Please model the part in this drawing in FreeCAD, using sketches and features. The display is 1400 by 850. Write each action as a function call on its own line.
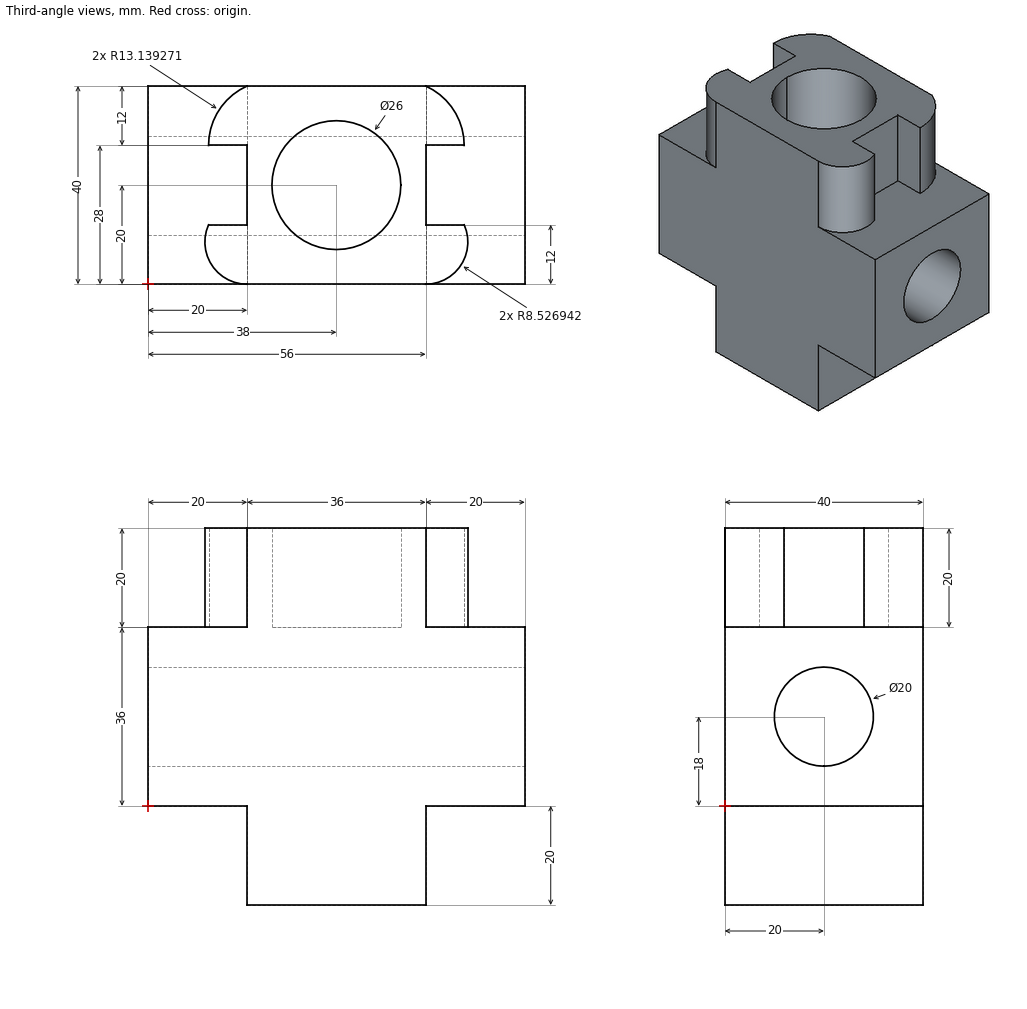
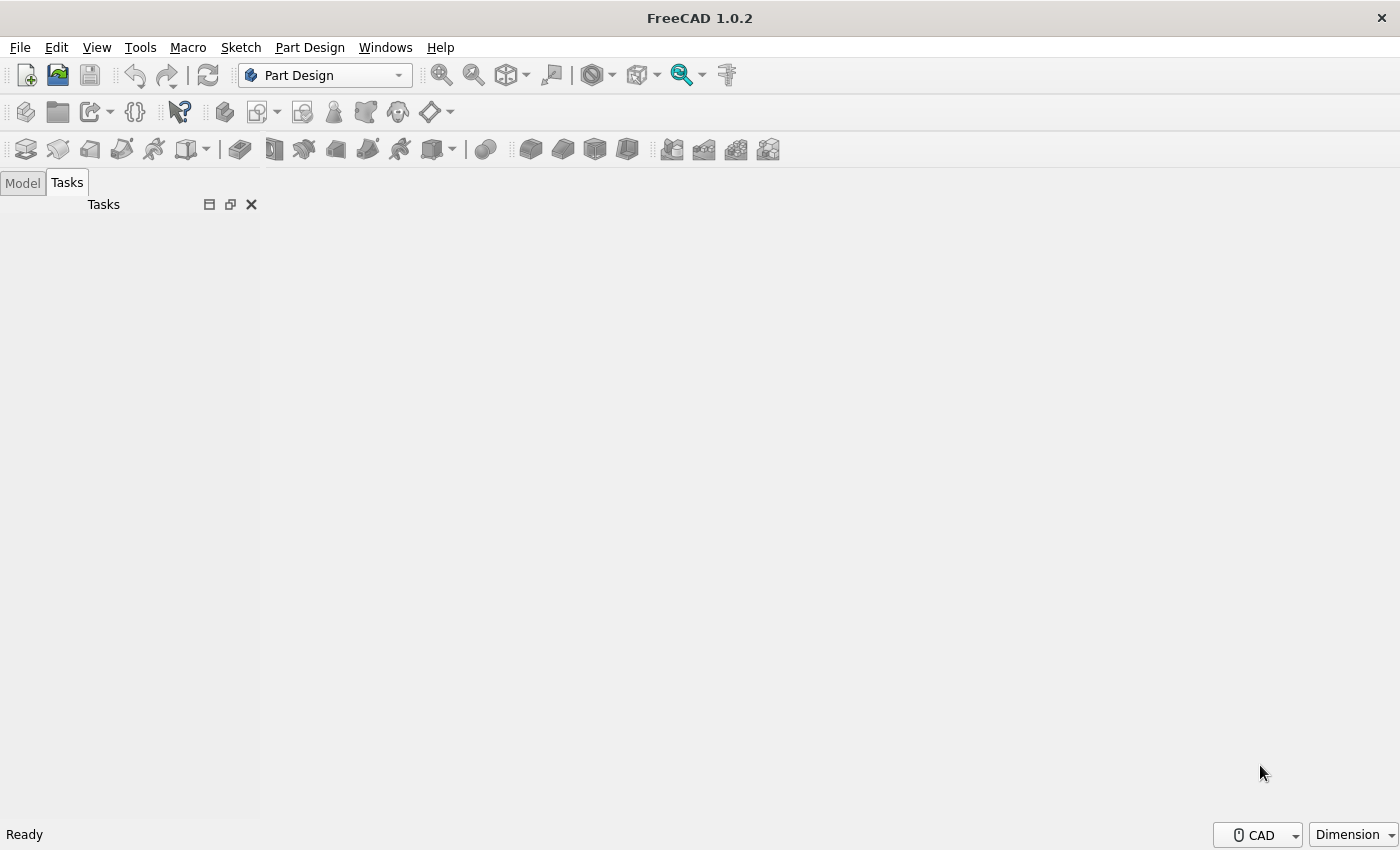
click(1032, 76)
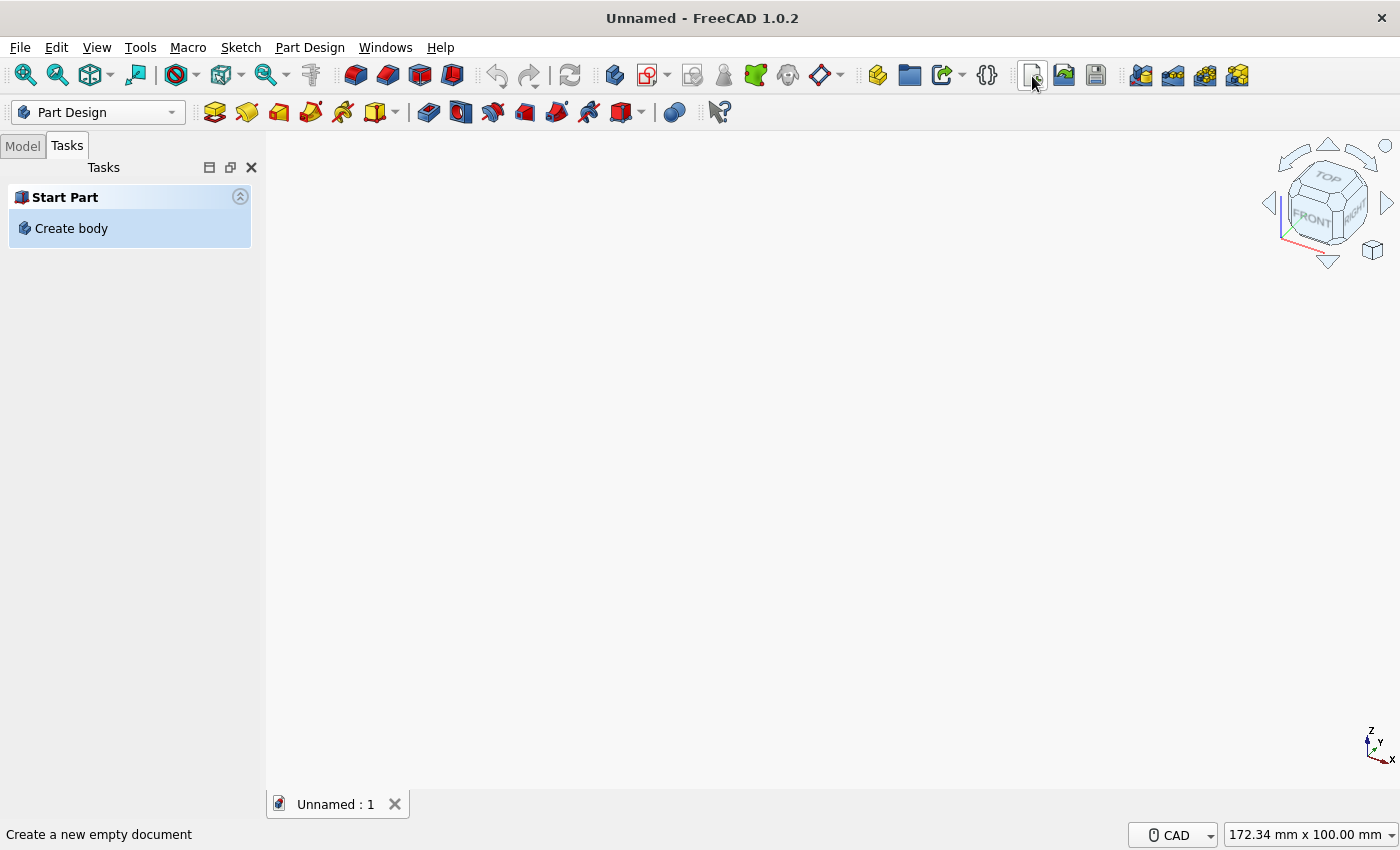
click(648, 76)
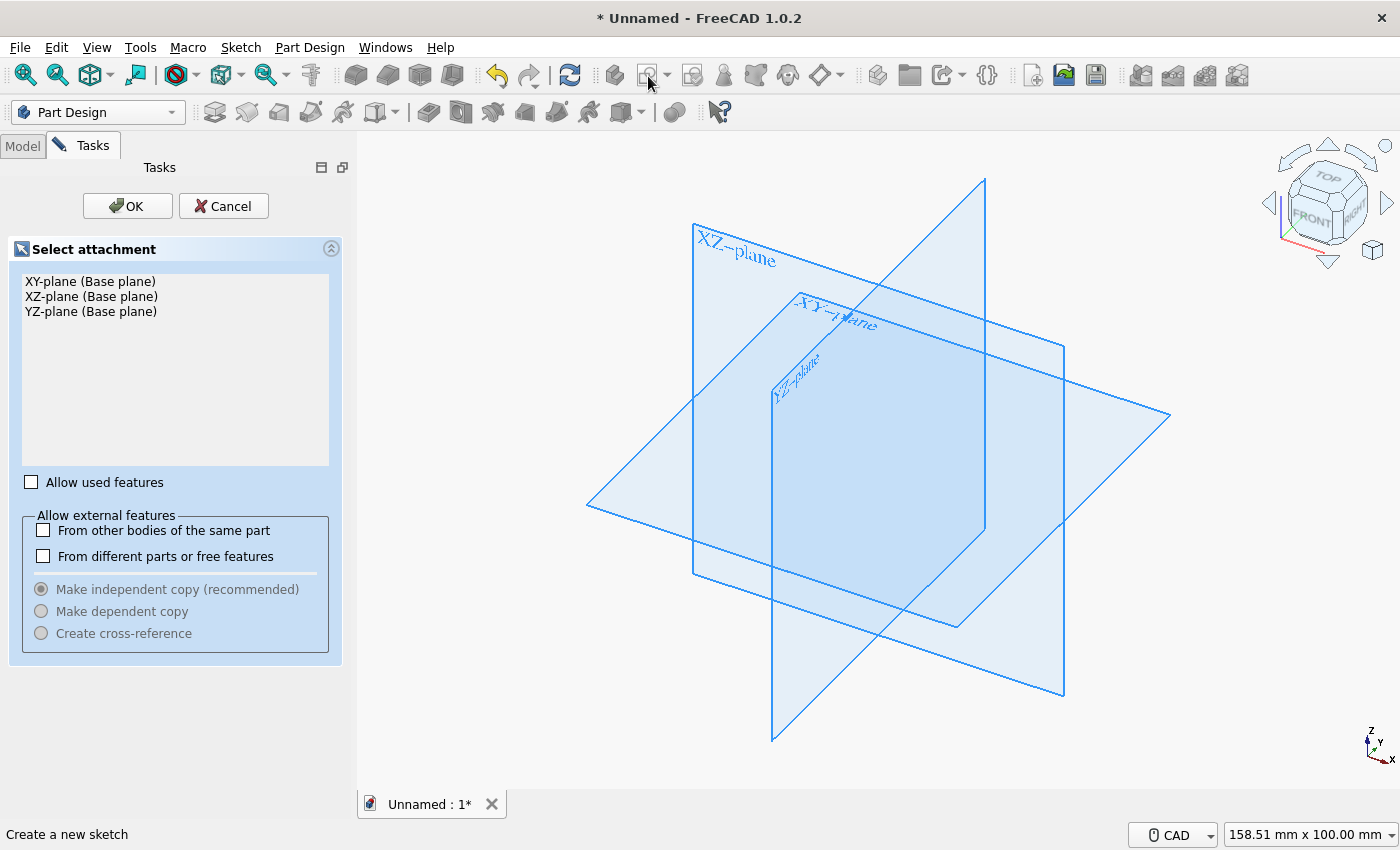
click(82, 296)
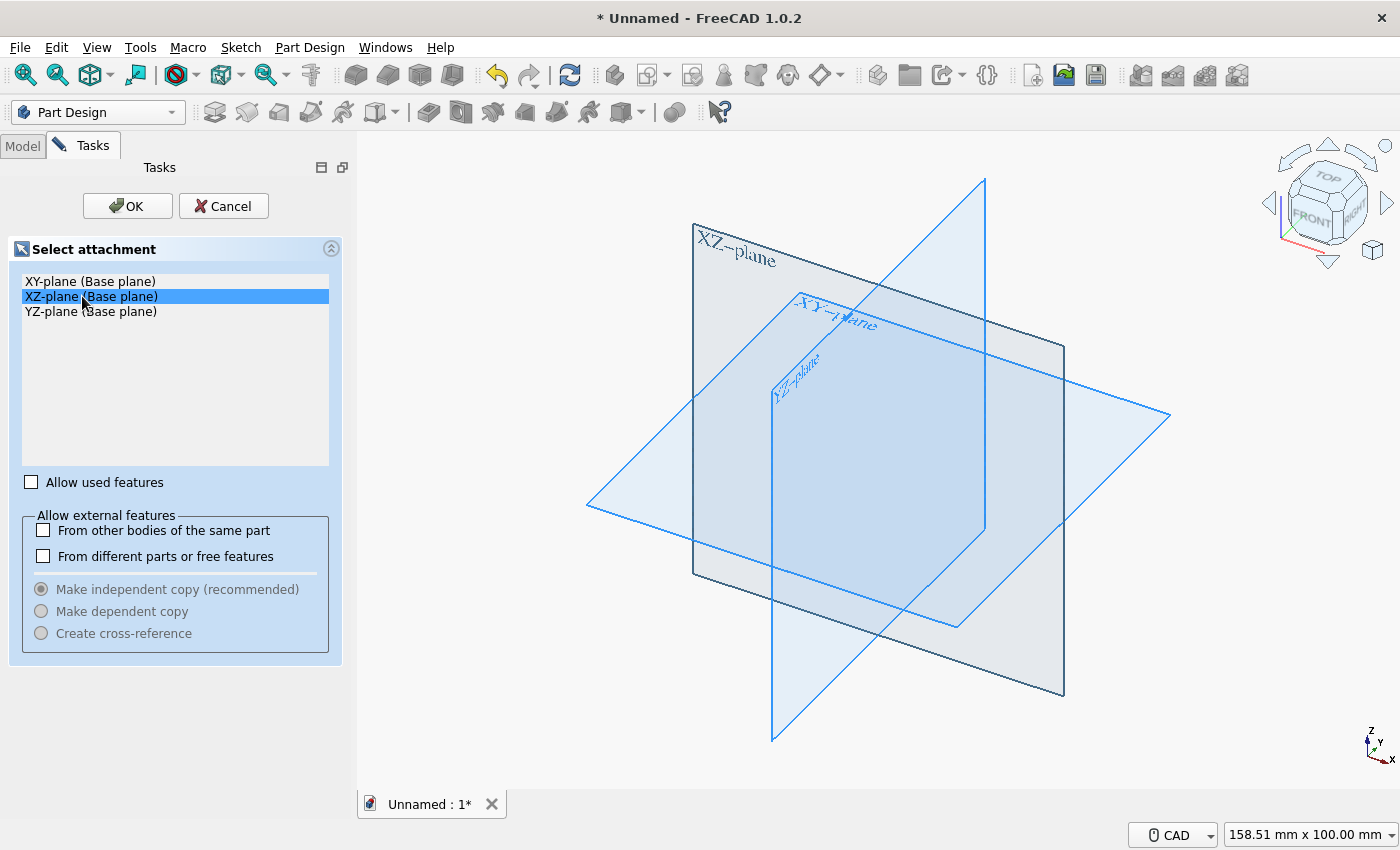
click(128, 206)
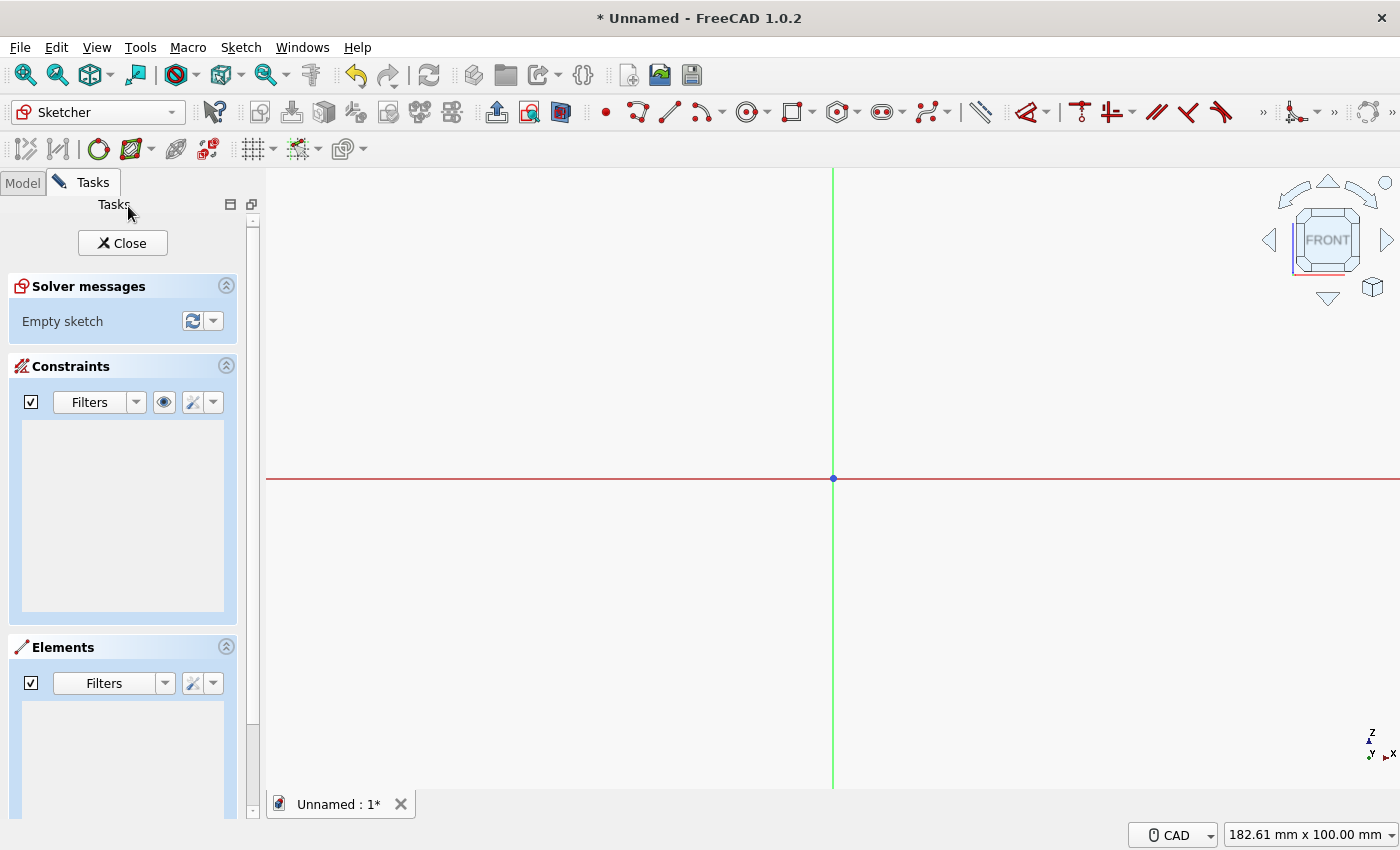
scroll(294, 761, down, 1)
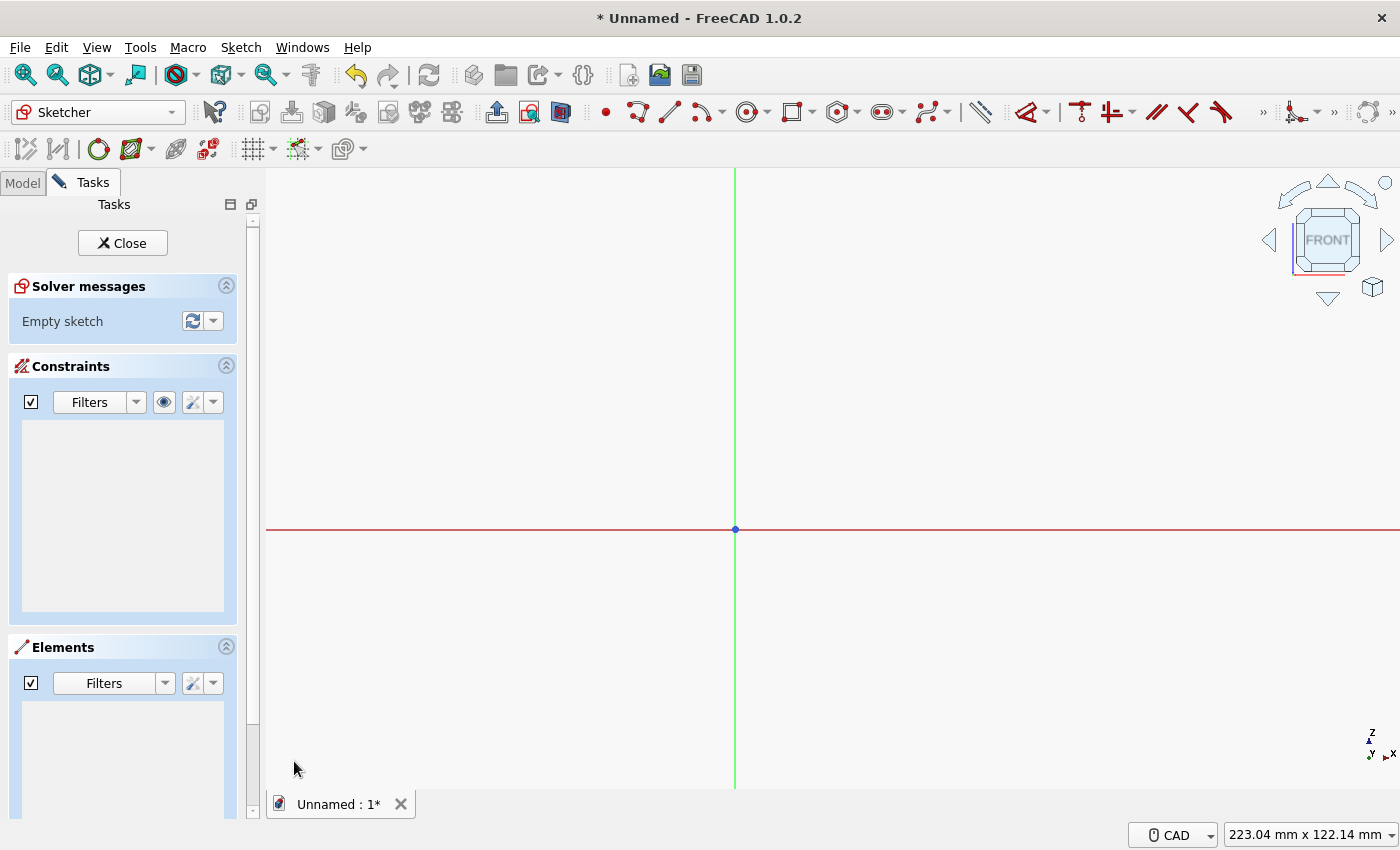
click(638, 112)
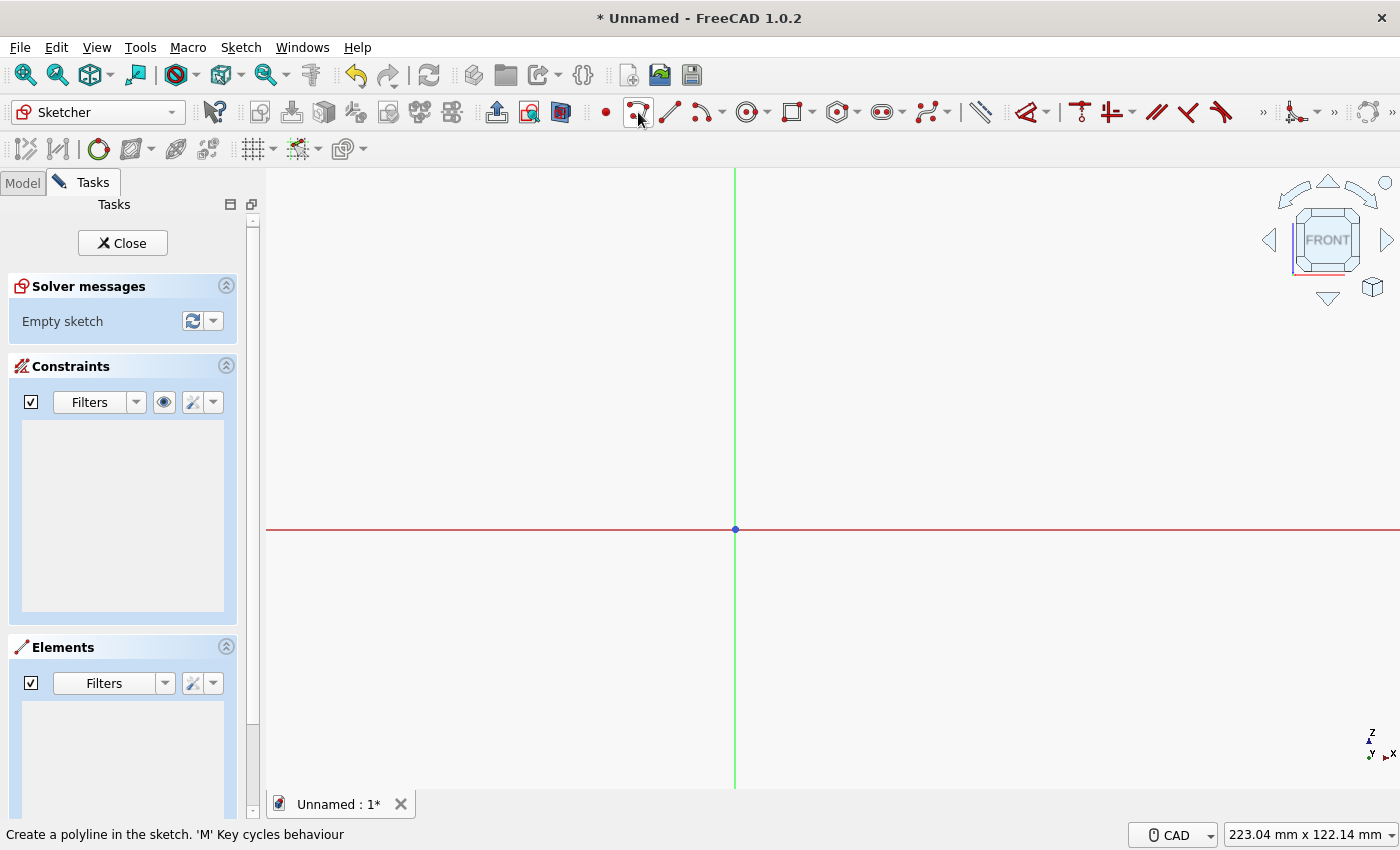
click(735, 530)
click(744, 347)
click(837, 347)
click(837, 245)
click(1020, 245)
click(1020, 347)
click(1122, 347)
click(1122, 530)
click(1020, 521)
click(1020, 632)
click(837, 632)
click(837, 521)
click(735, 530)
key(Escape)
key(Escape)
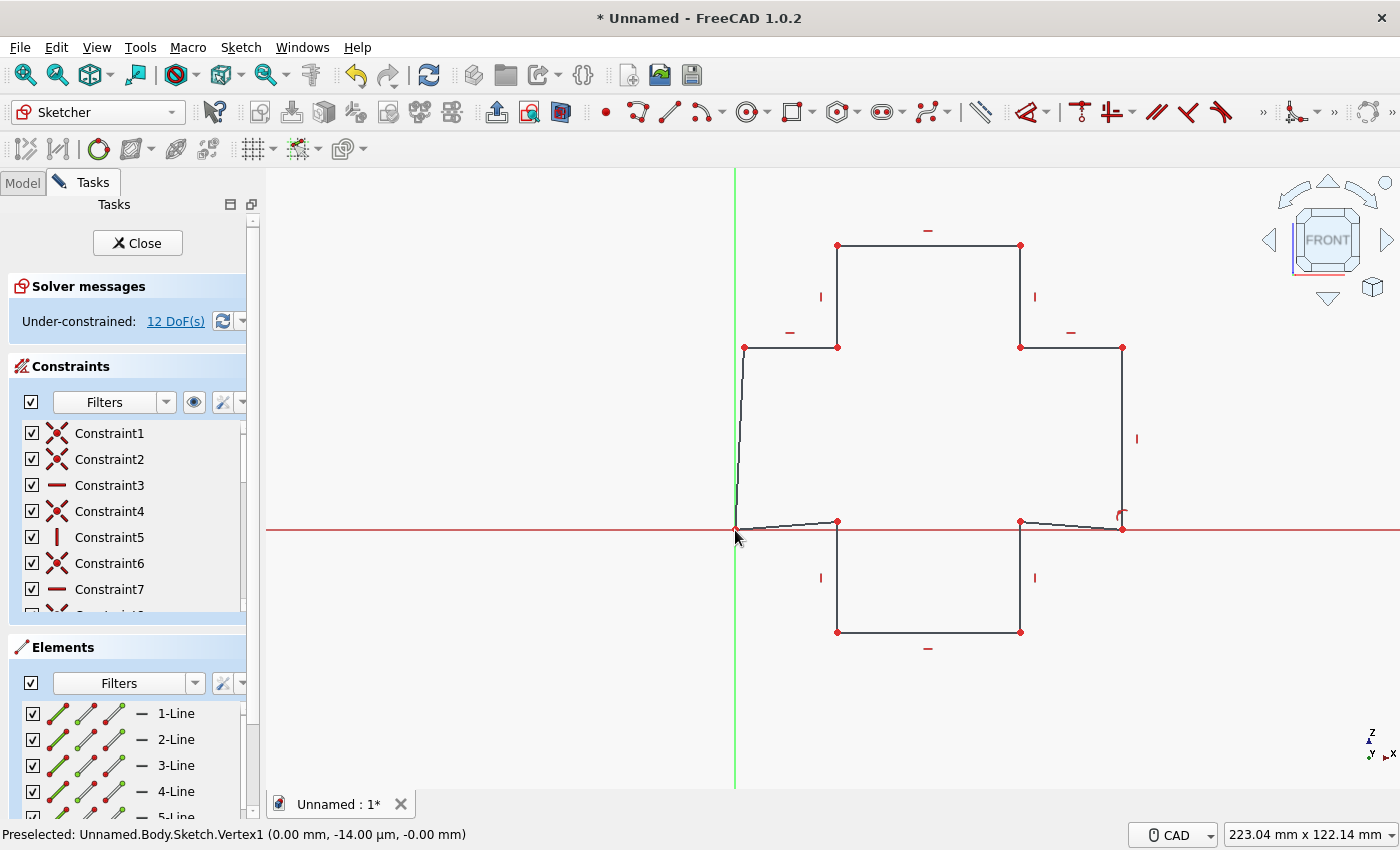
click(738, 475)